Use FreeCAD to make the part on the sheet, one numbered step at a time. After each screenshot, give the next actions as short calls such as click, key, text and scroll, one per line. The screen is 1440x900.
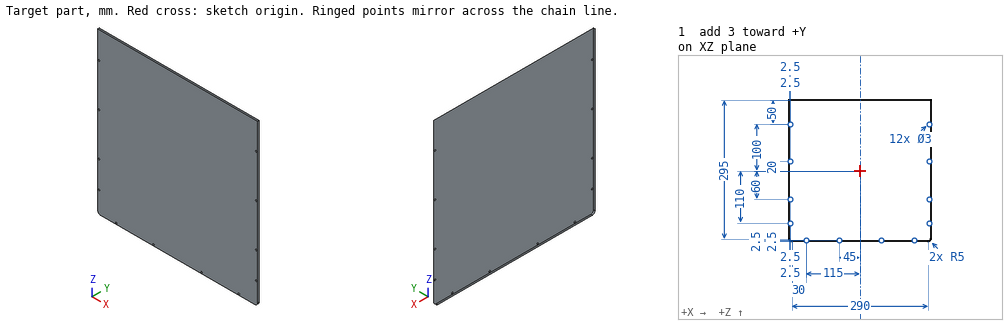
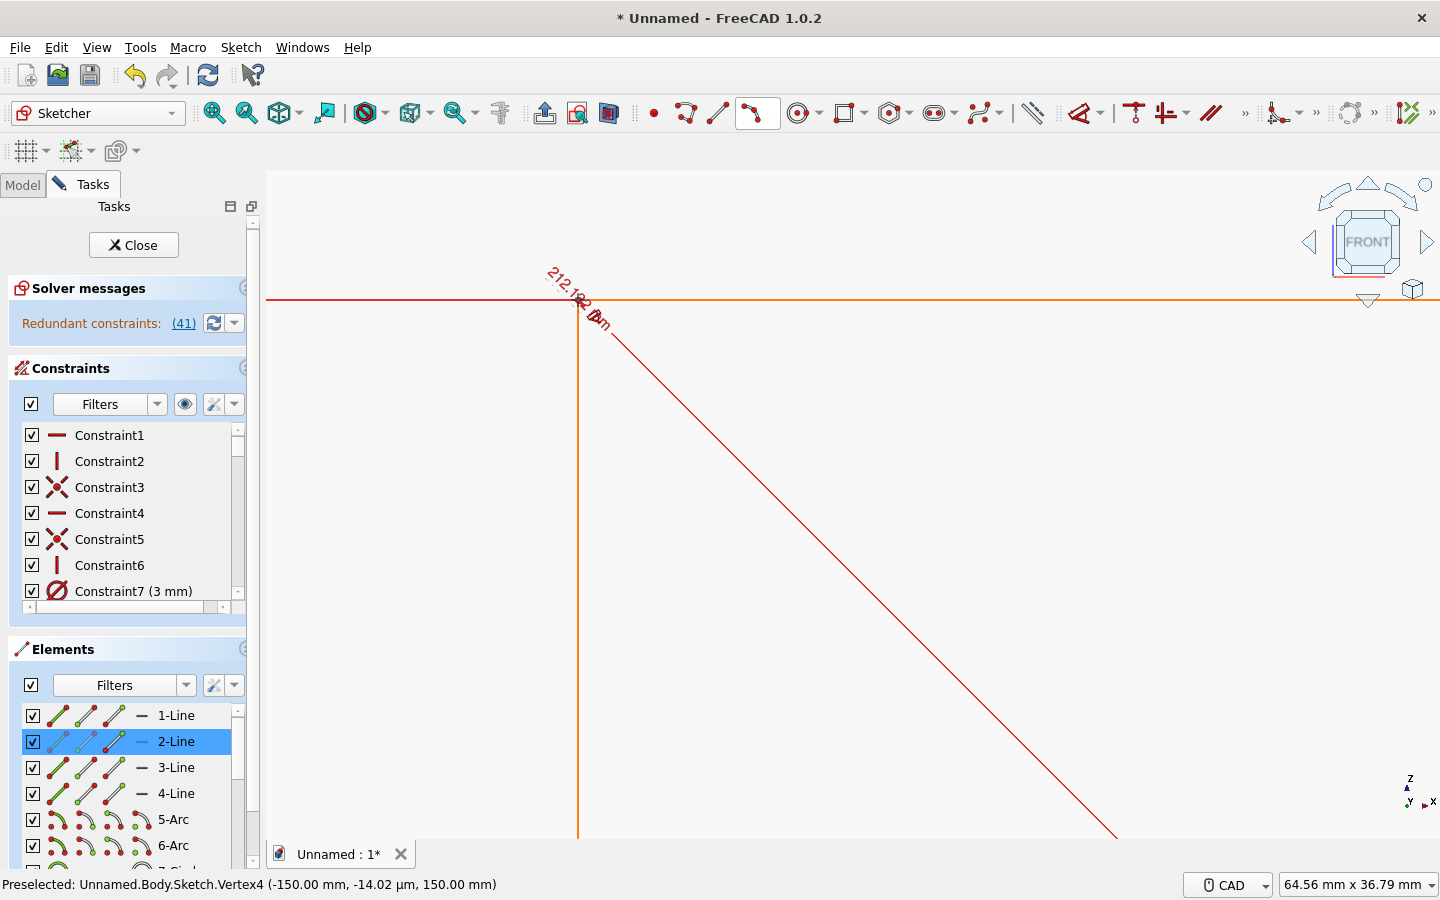
scroll(582, 302, down, 13)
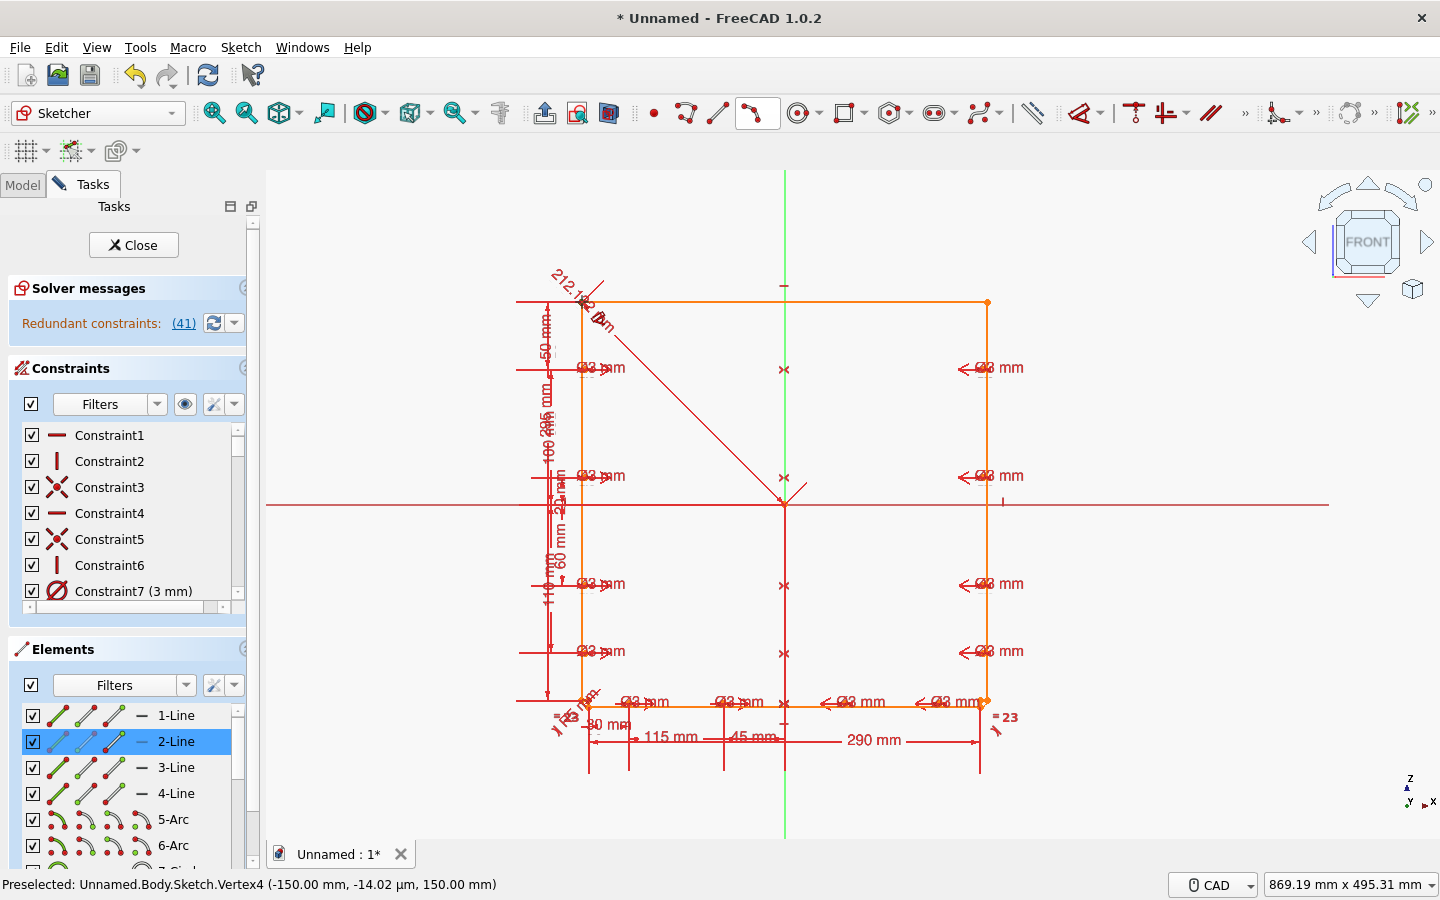
scroll(585, 370, up, 13)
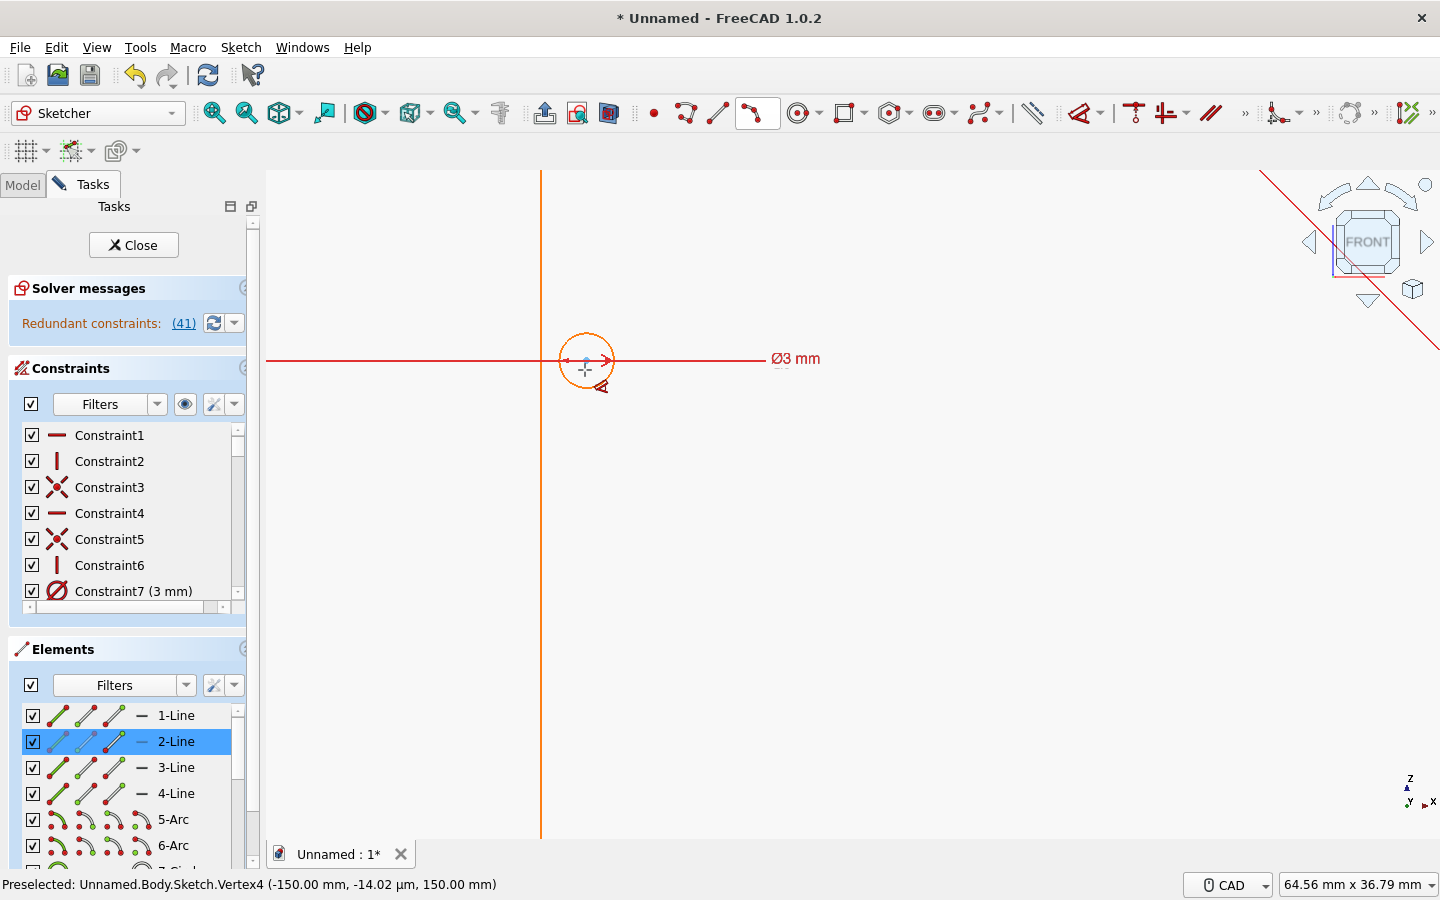
click(587, 361)
click(564, 395)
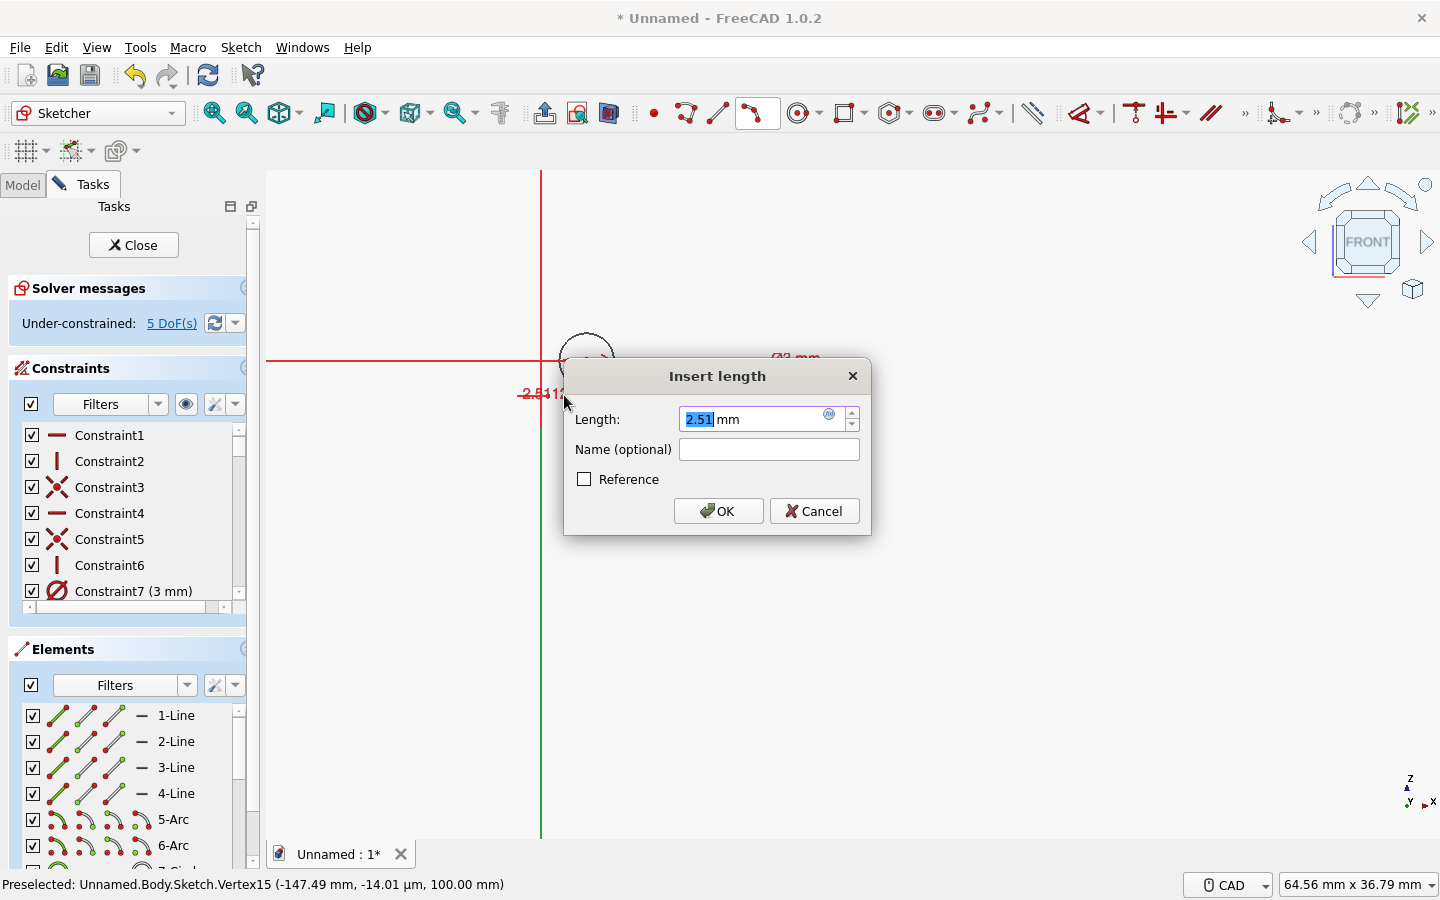
text(2.5)
key(Return)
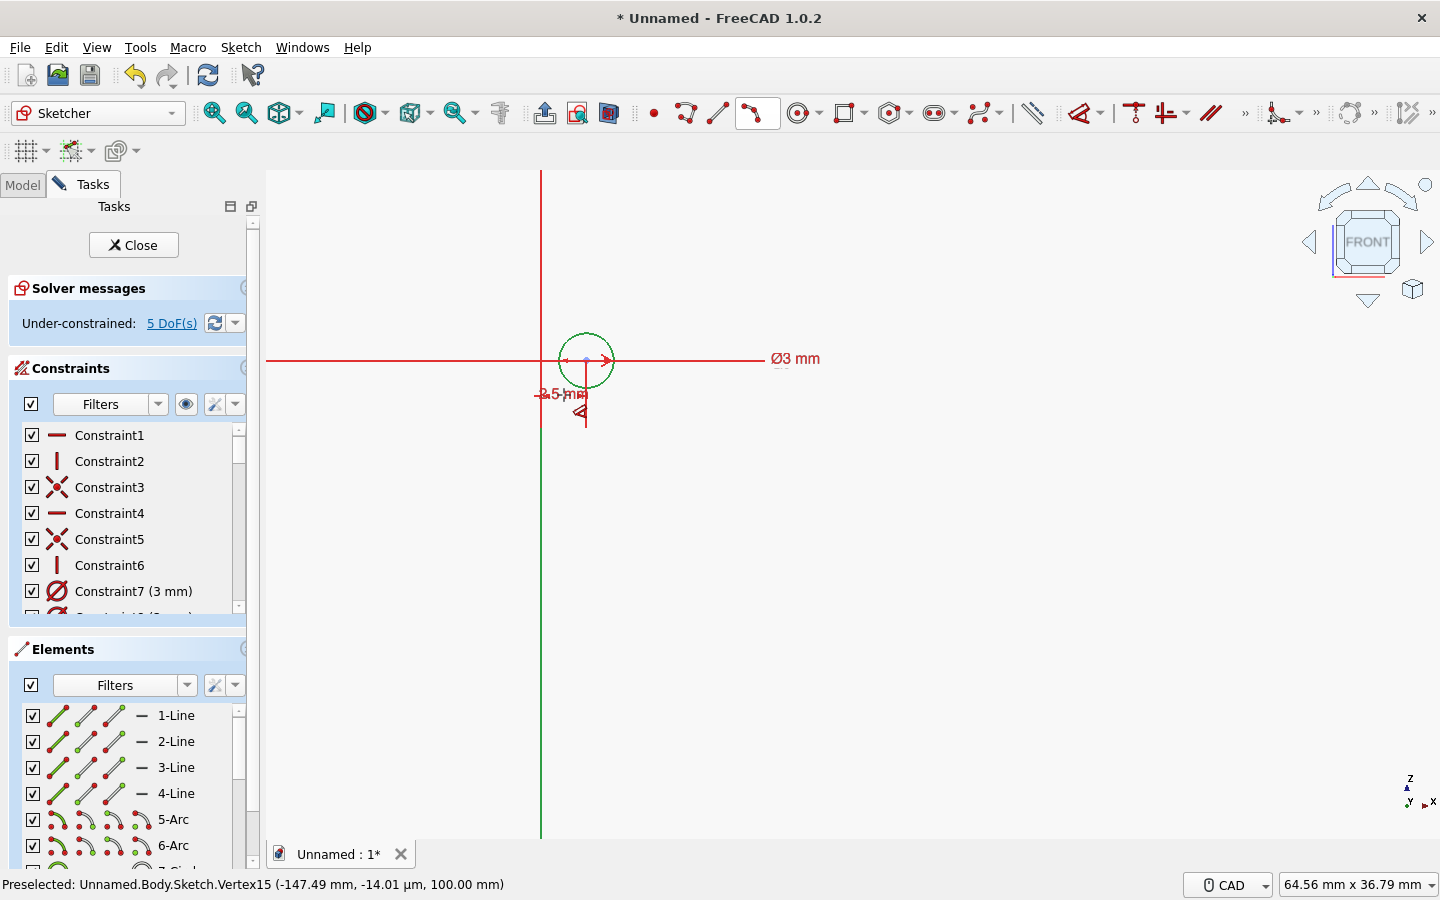
scroll(585, 370, down, 13)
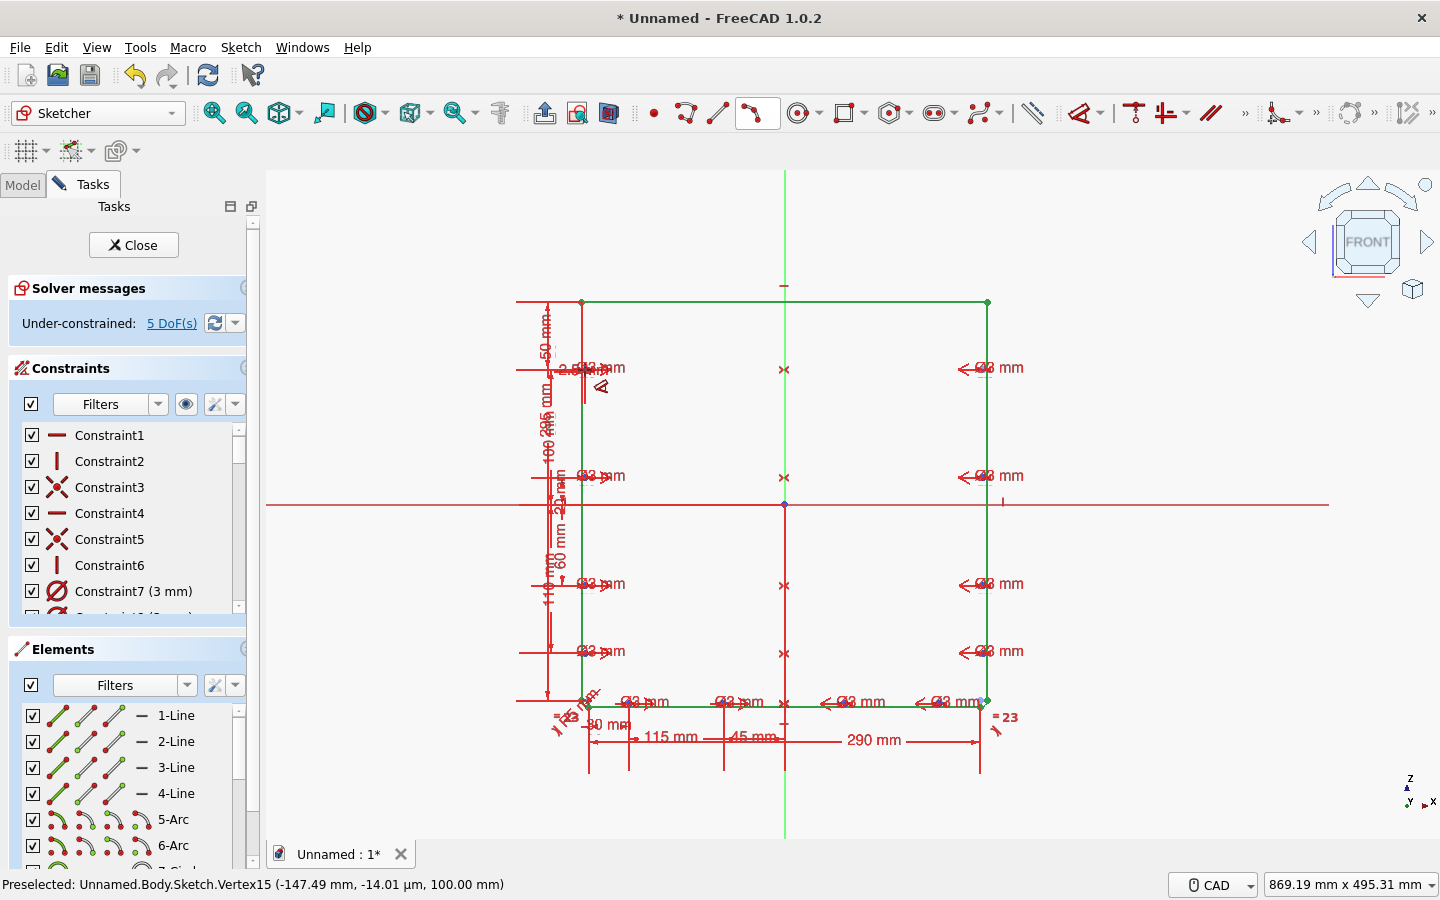
scroll(582, 302, up, 13)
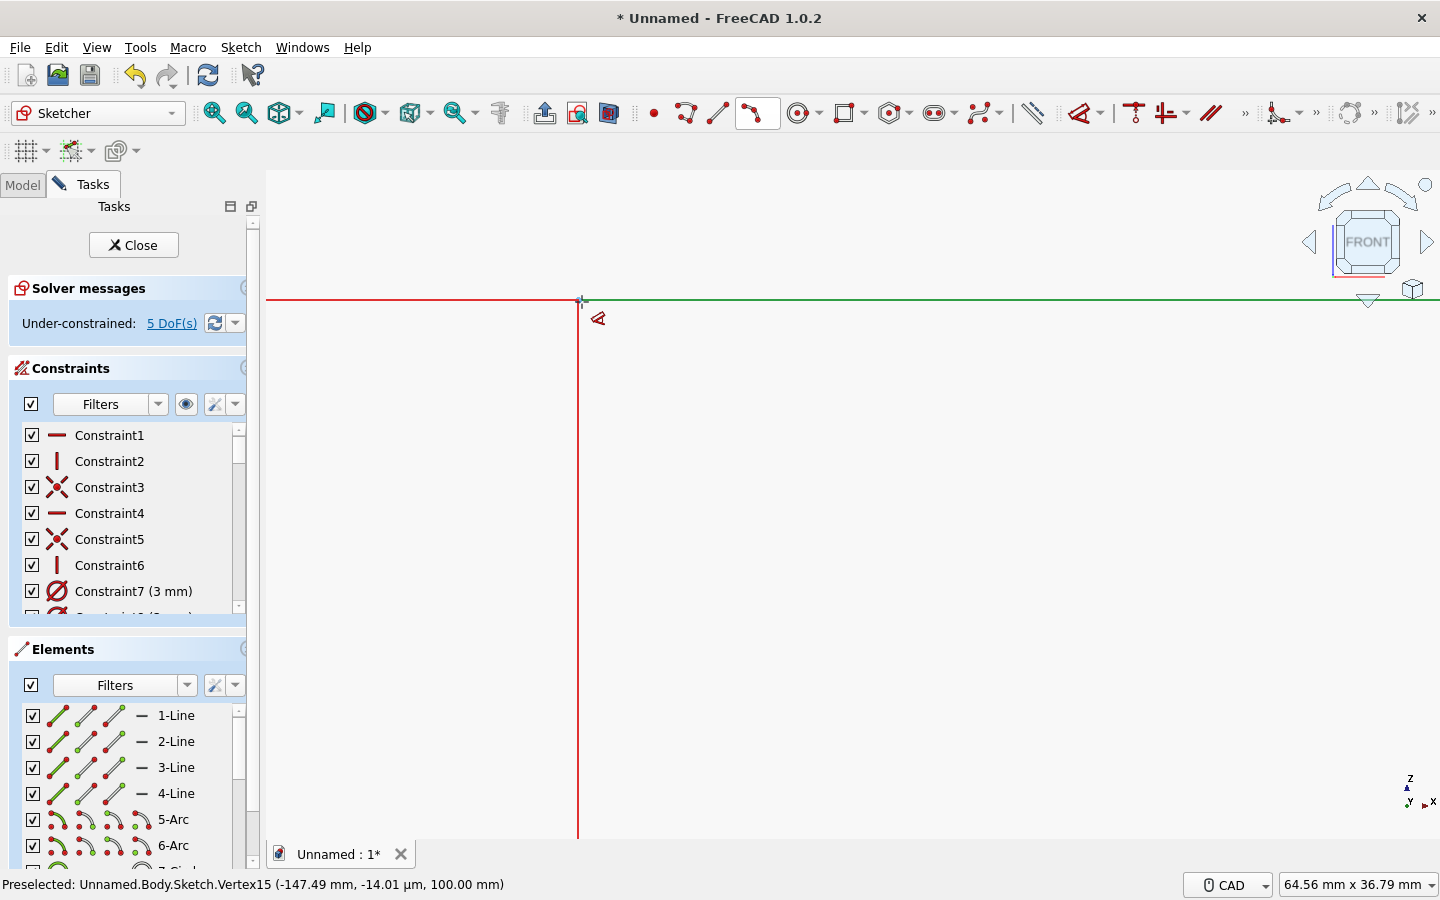
click(578, 300)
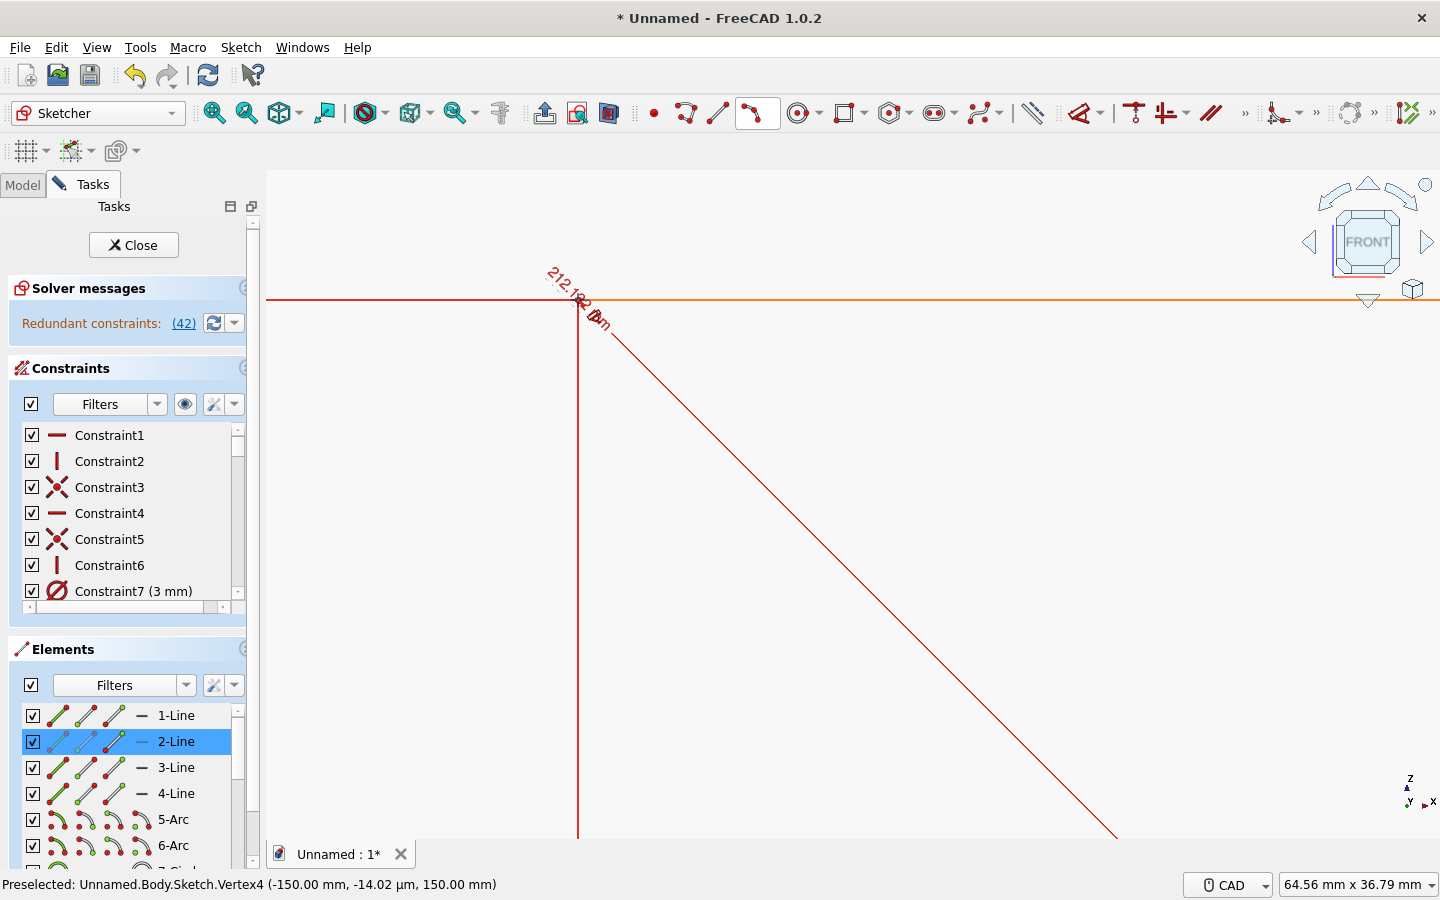
scroll(582, 302, down, 13)